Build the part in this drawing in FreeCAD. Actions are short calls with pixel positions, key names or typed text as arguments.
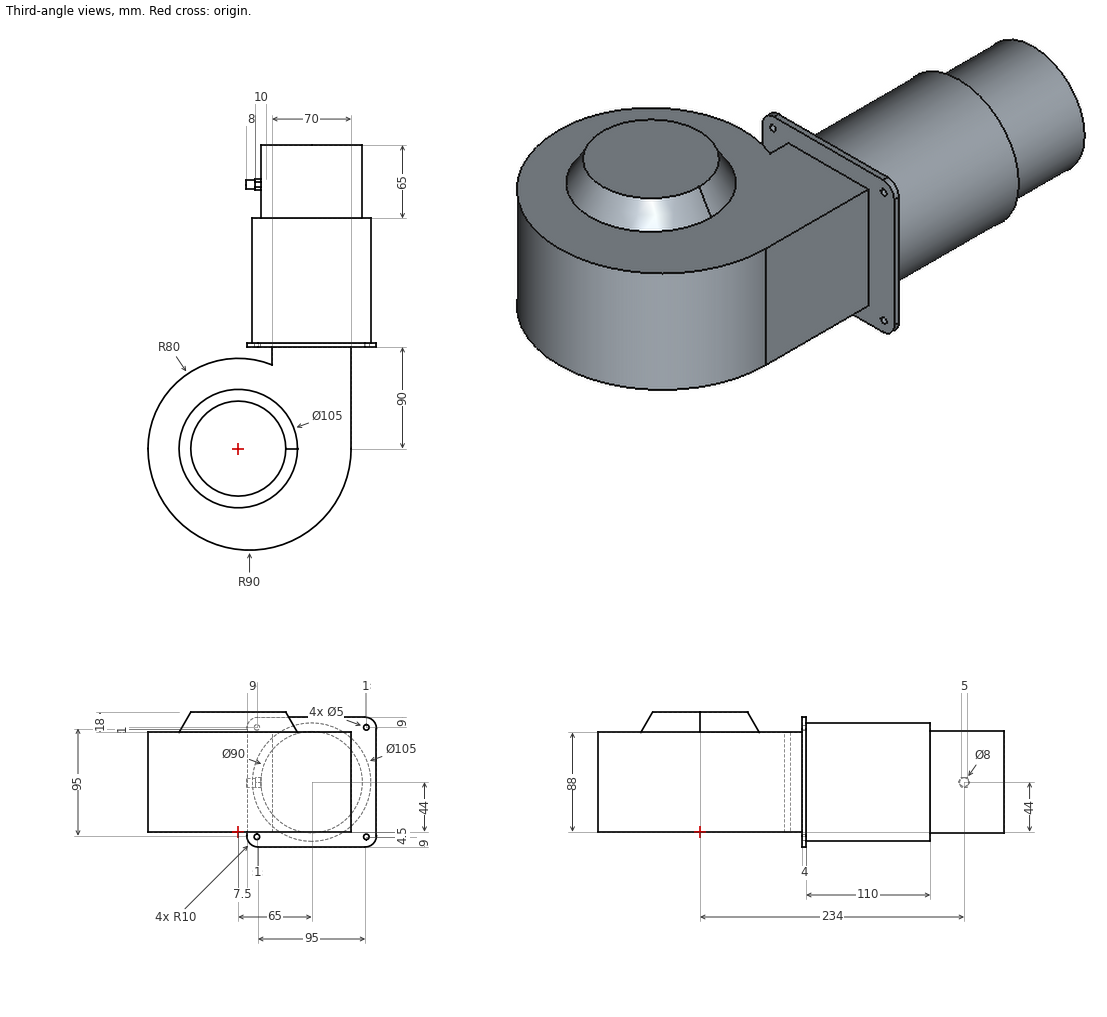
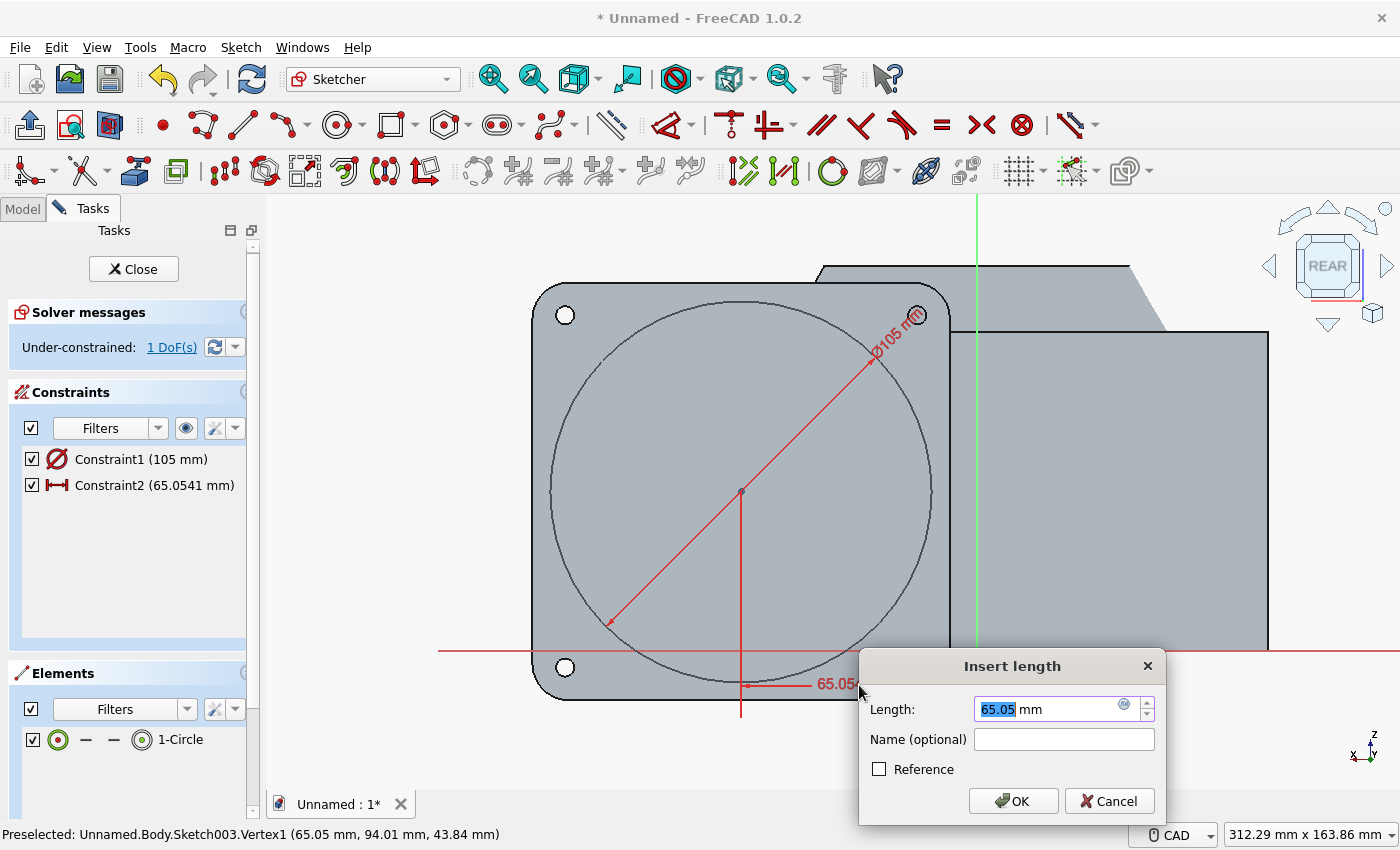
text(65)
key(Return)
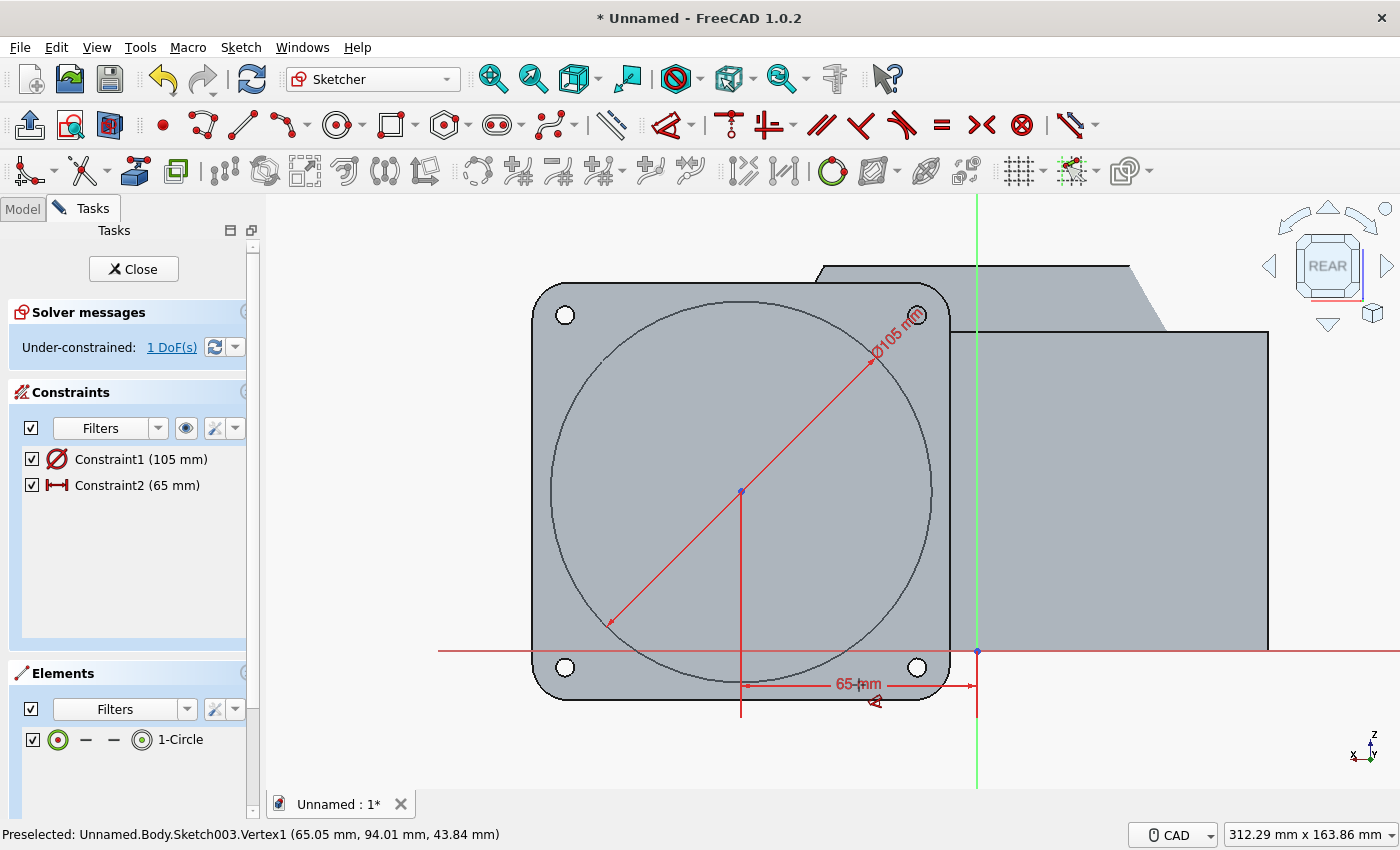
click(741, 492)
click(1011, 572)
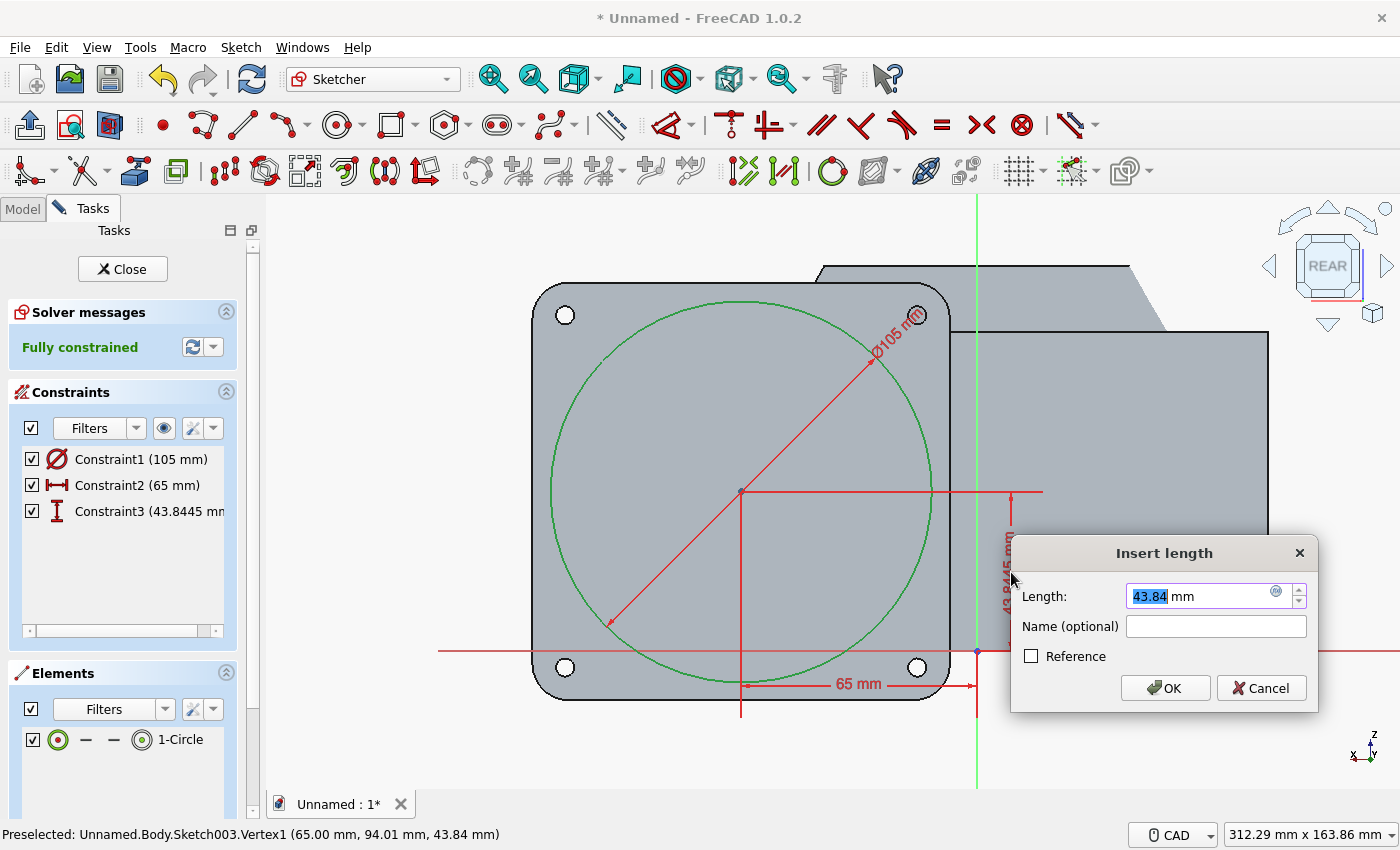
text(44)
key(Return)
key(Escape)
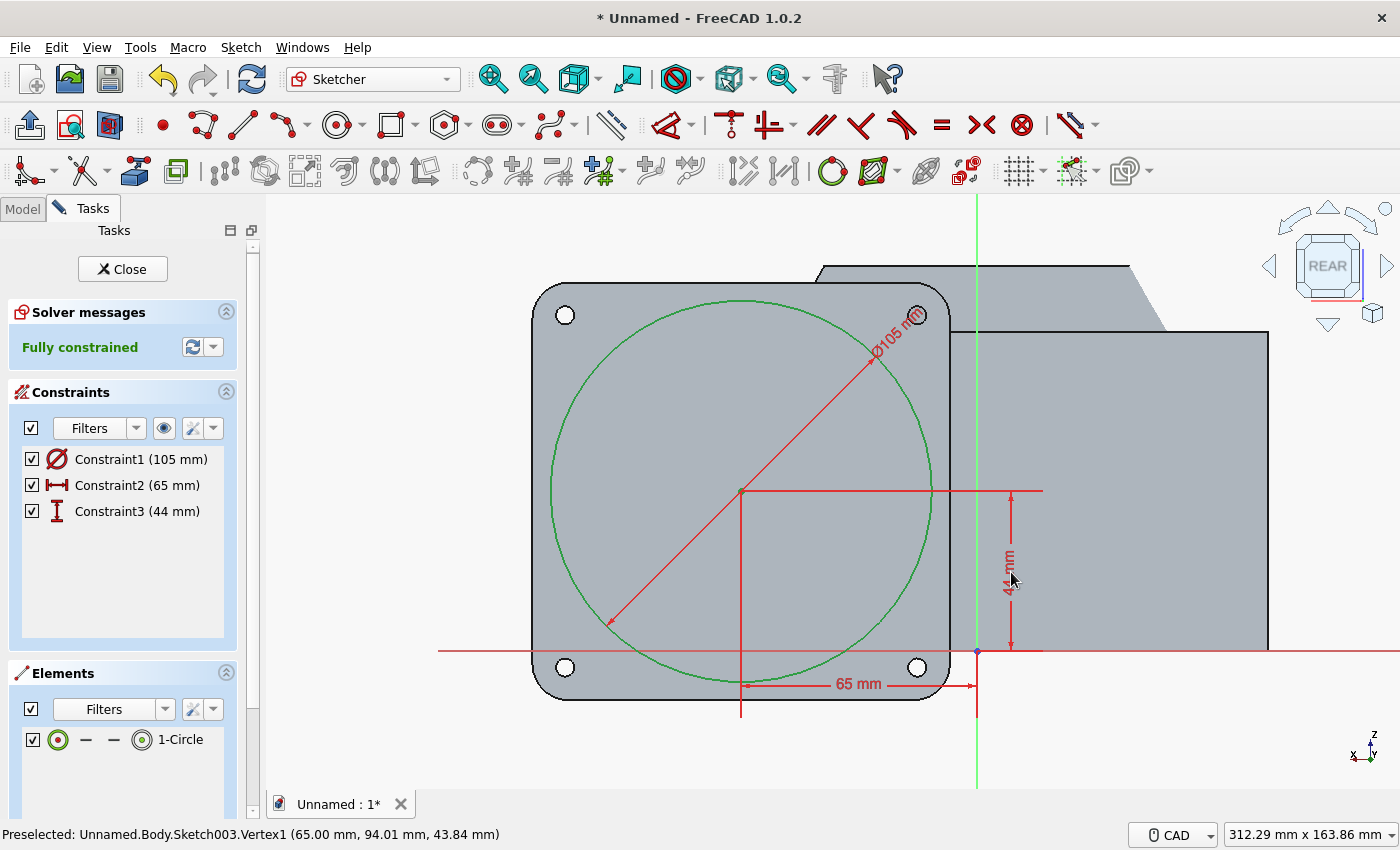
click(123, 269)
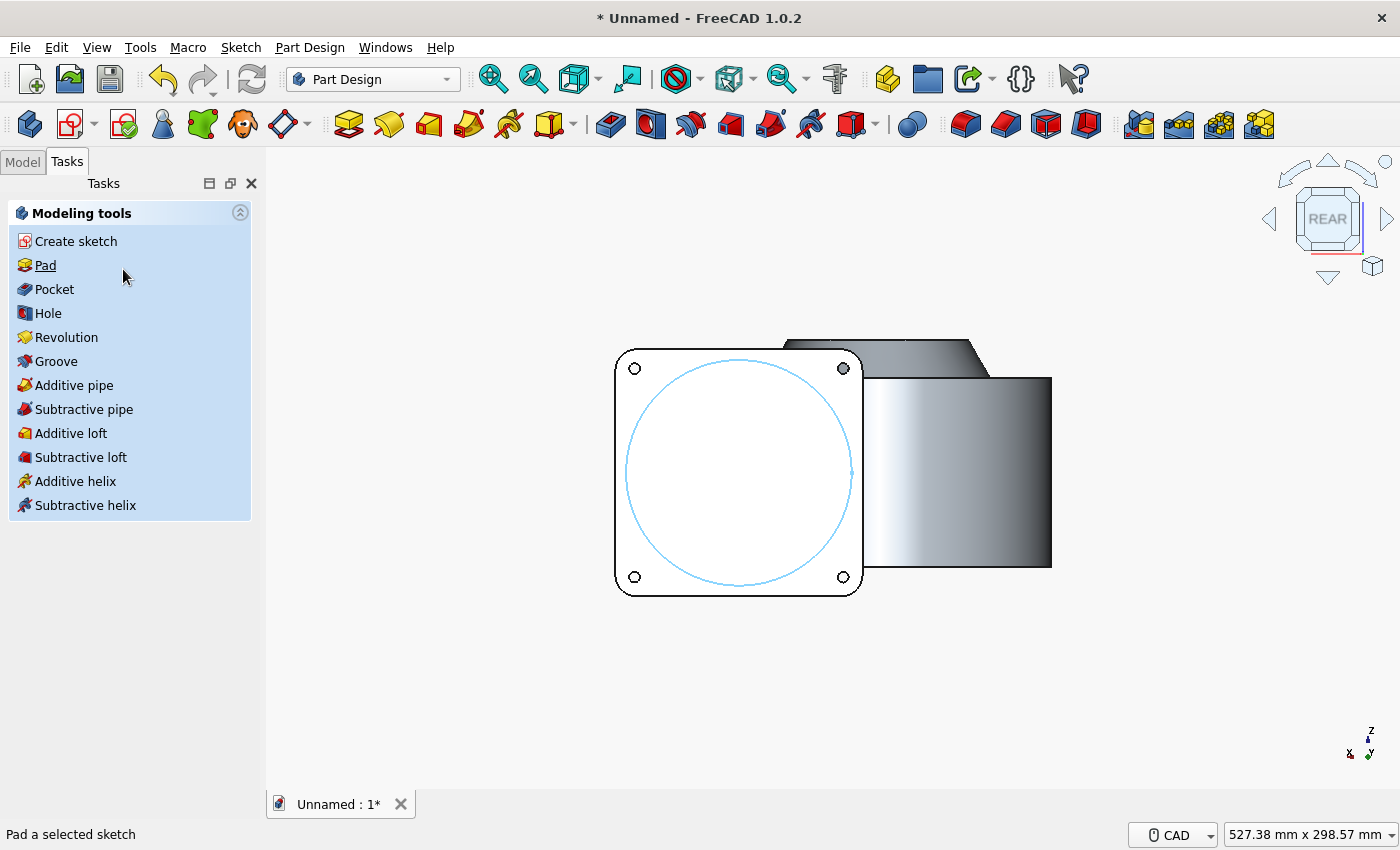
click(350, 124)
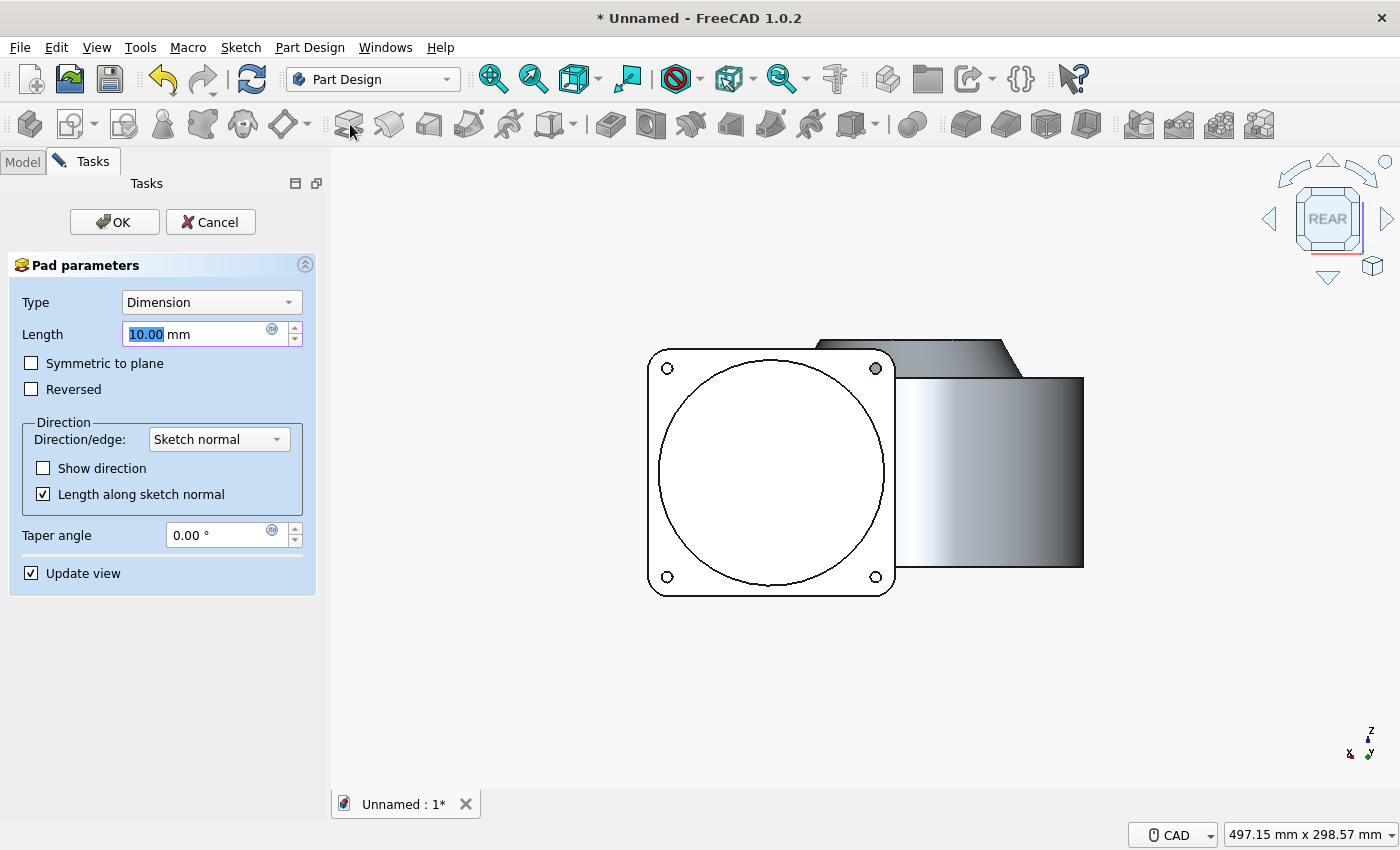
text(110)
key(Tab)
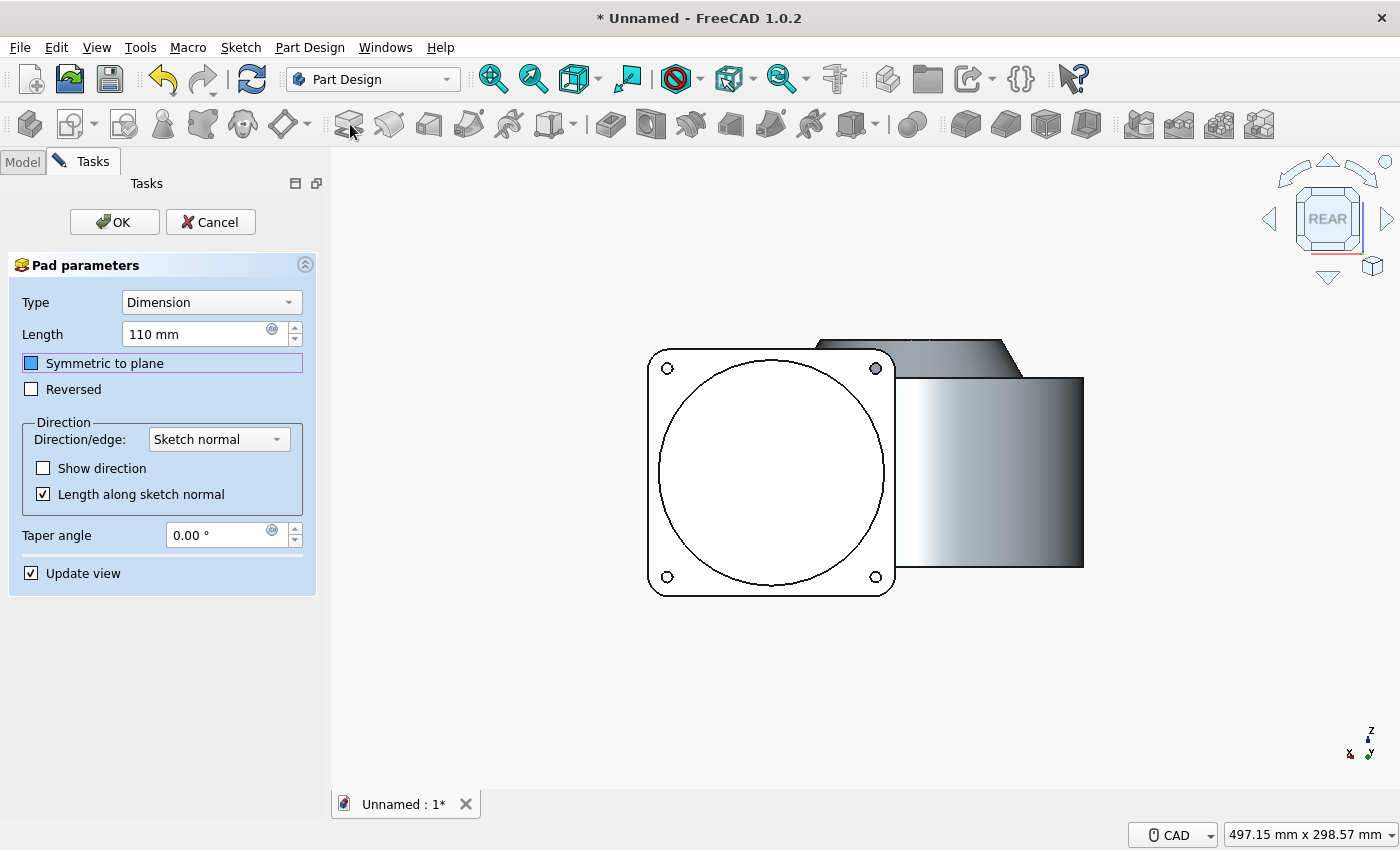
click(115, 222)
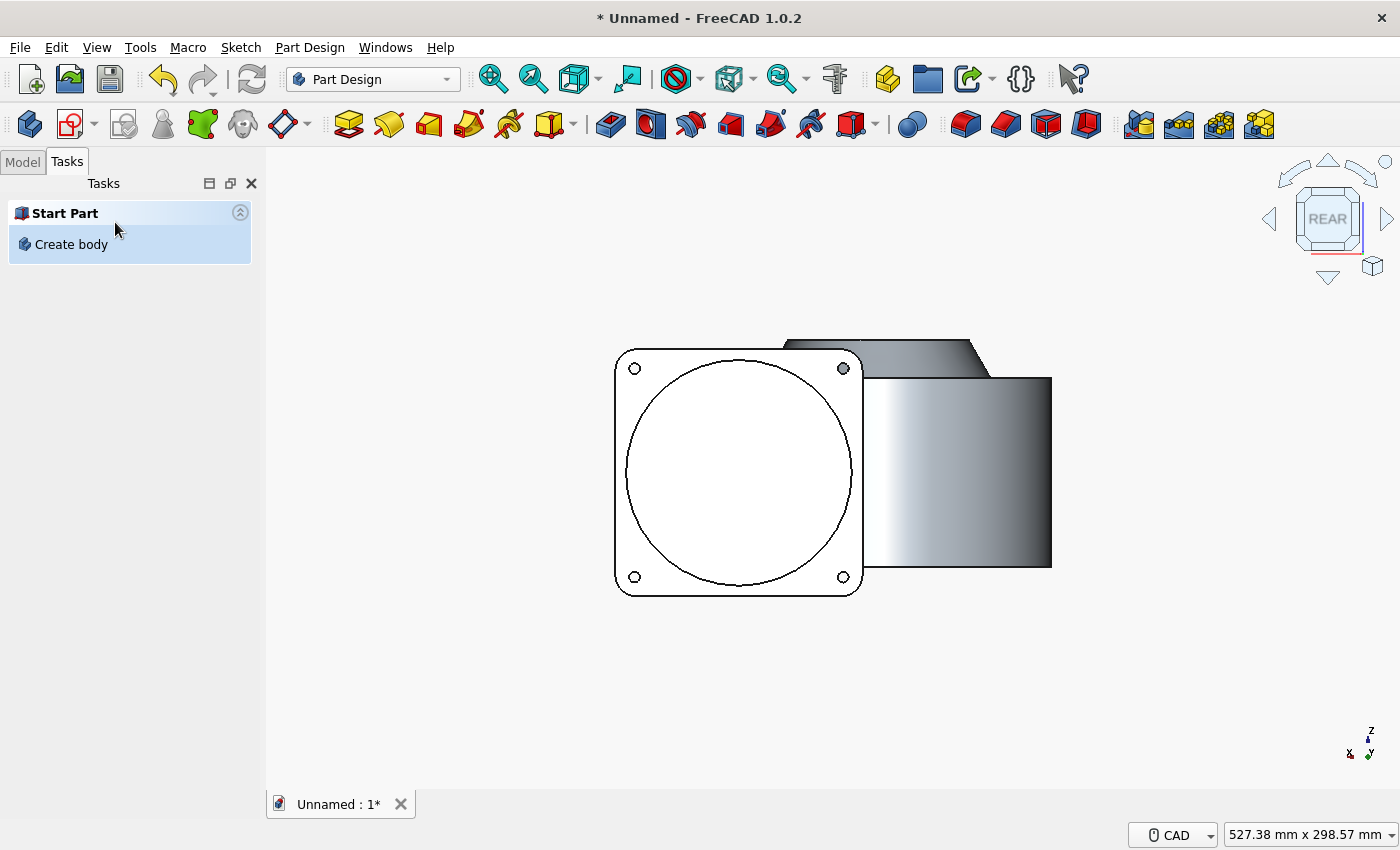
click(494, 80)